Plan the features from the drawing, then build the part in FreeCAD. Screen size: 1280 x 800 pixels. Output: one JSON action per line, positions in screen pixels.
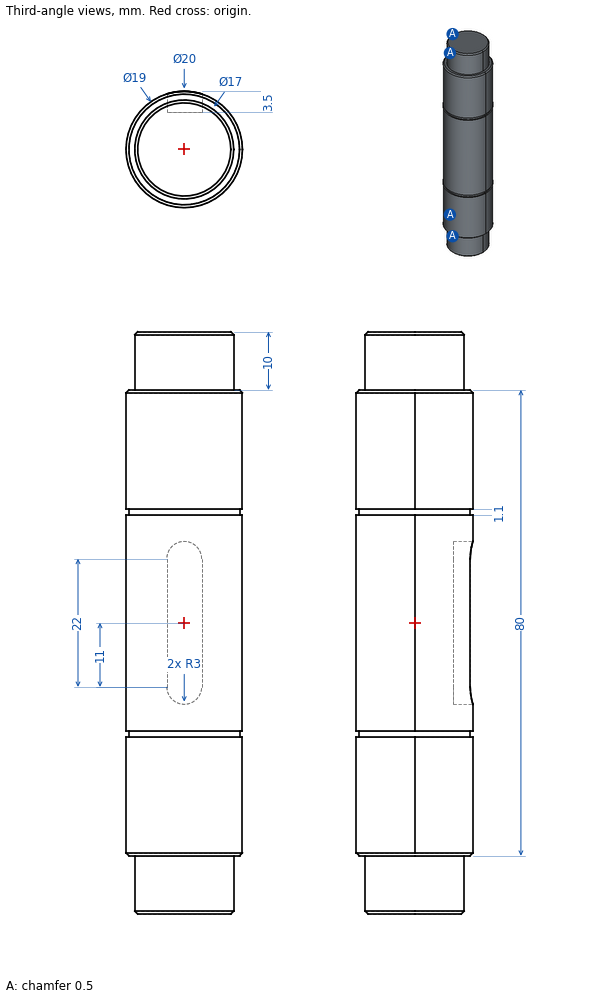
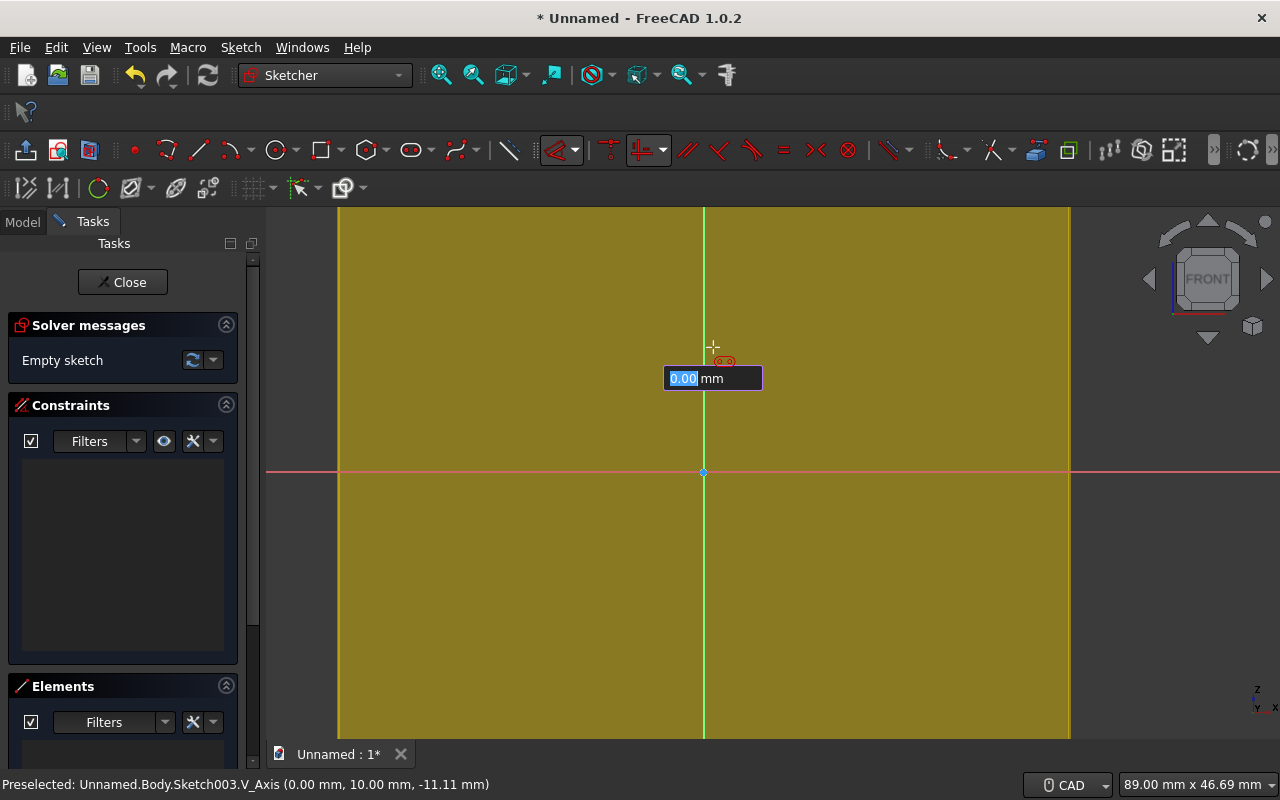
{"action": "left_click", "coordinate": [738, 435]}
{"action": "key", "text": "Escape"}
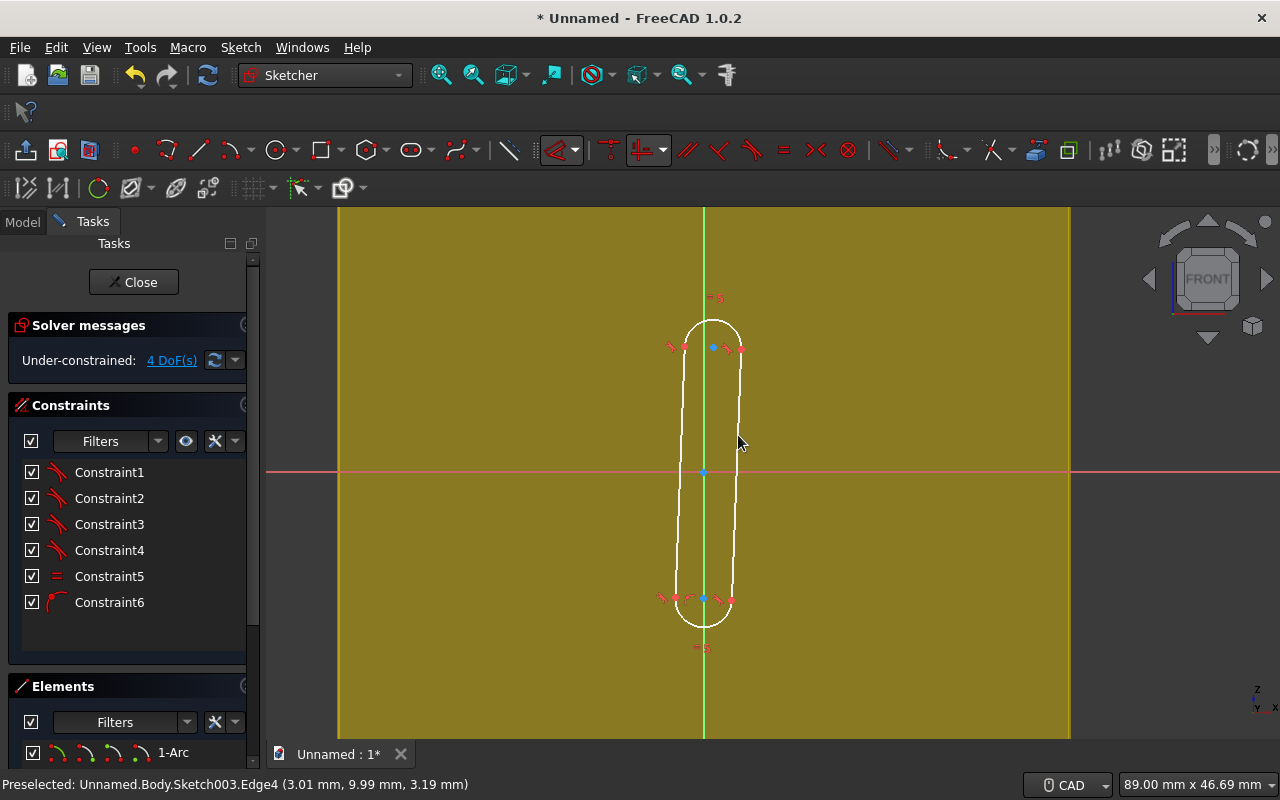
{"action": "left_click", "coordinate": [678, 523]}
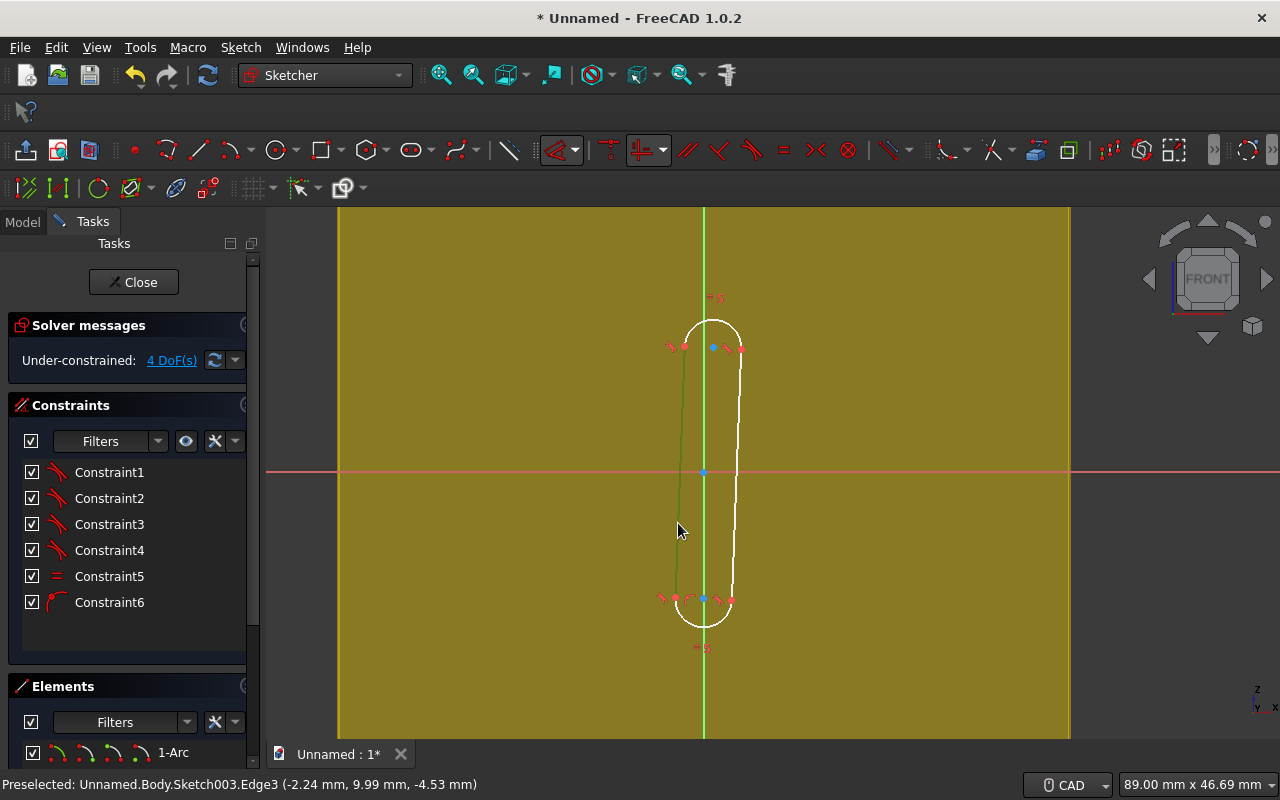
{"action": "left_click", "coordinate": [666, 150]}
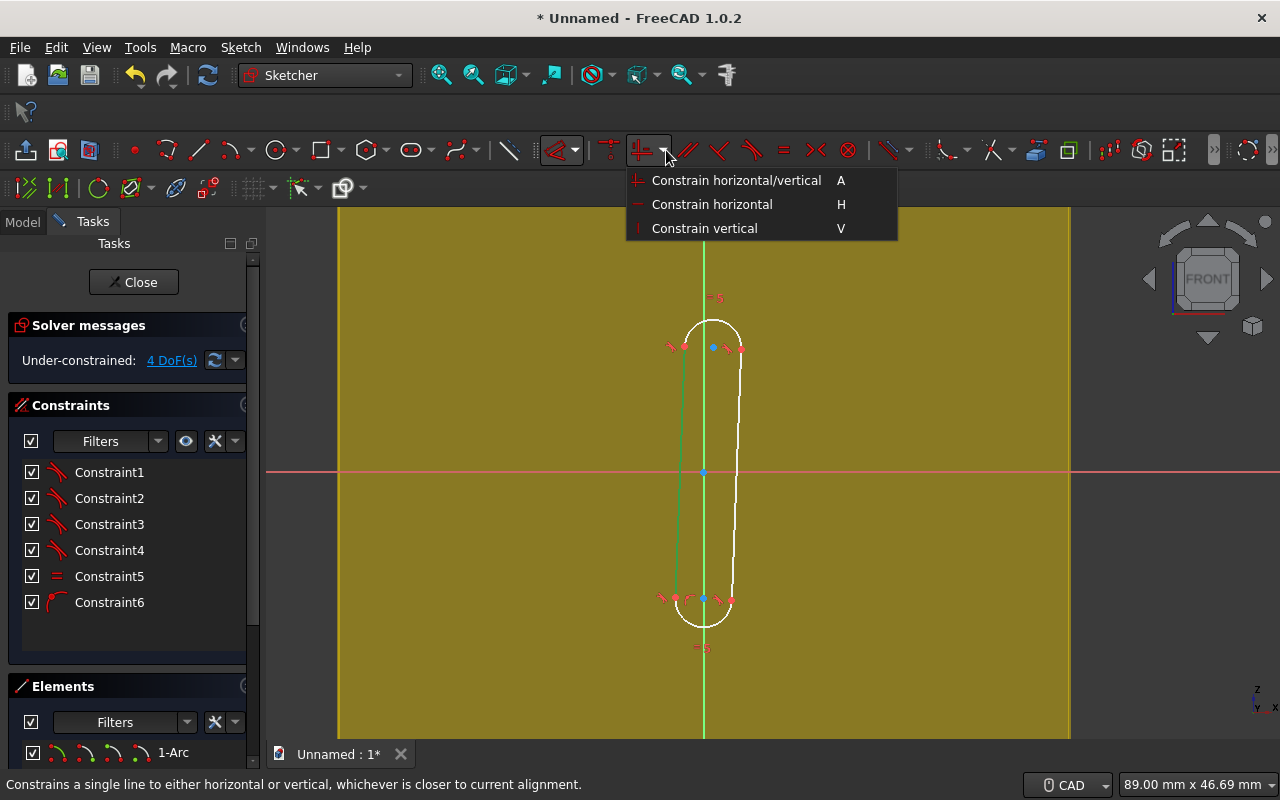
{"action": "left_click", "coordinate": [762, 228]}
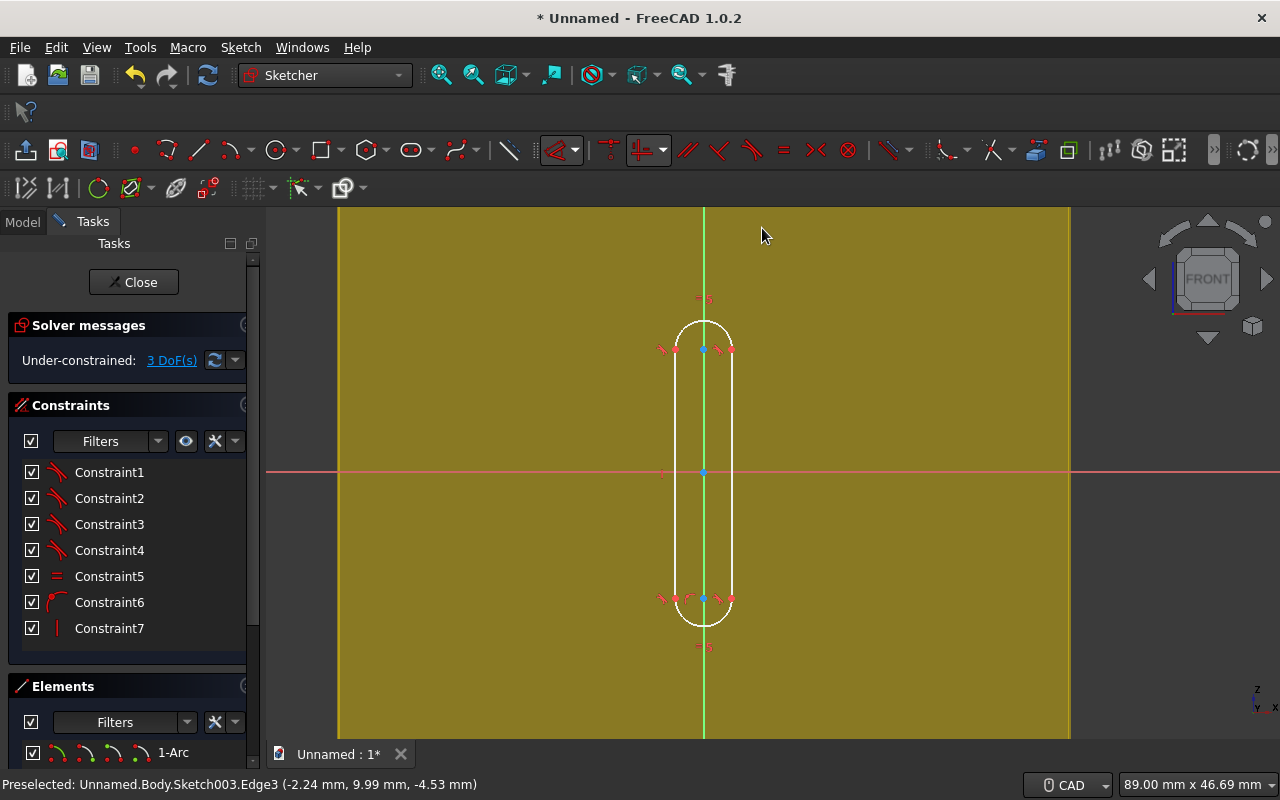
{"action": "key", "text": "d"}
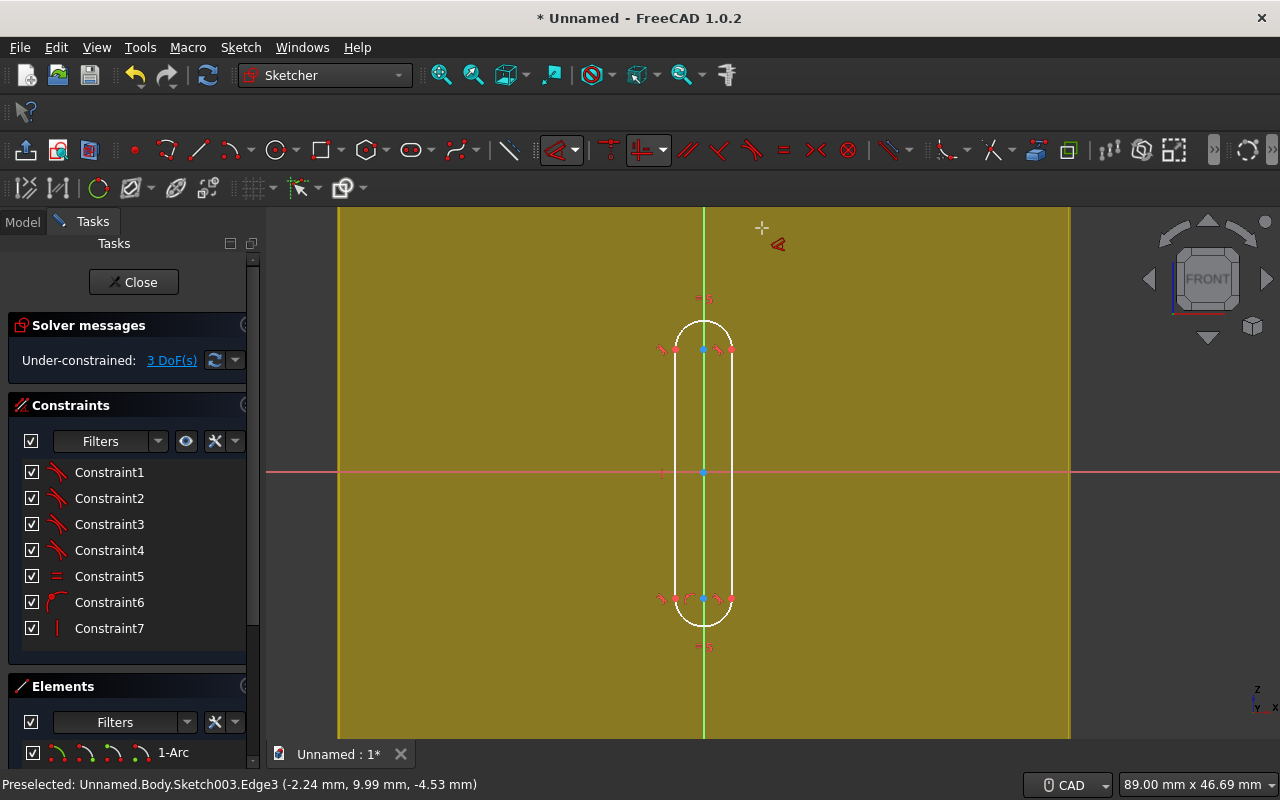
{"action": "left_click", "coordinate": [687, 621]}
{"action": "left_click", "coordinate": [668, 647]}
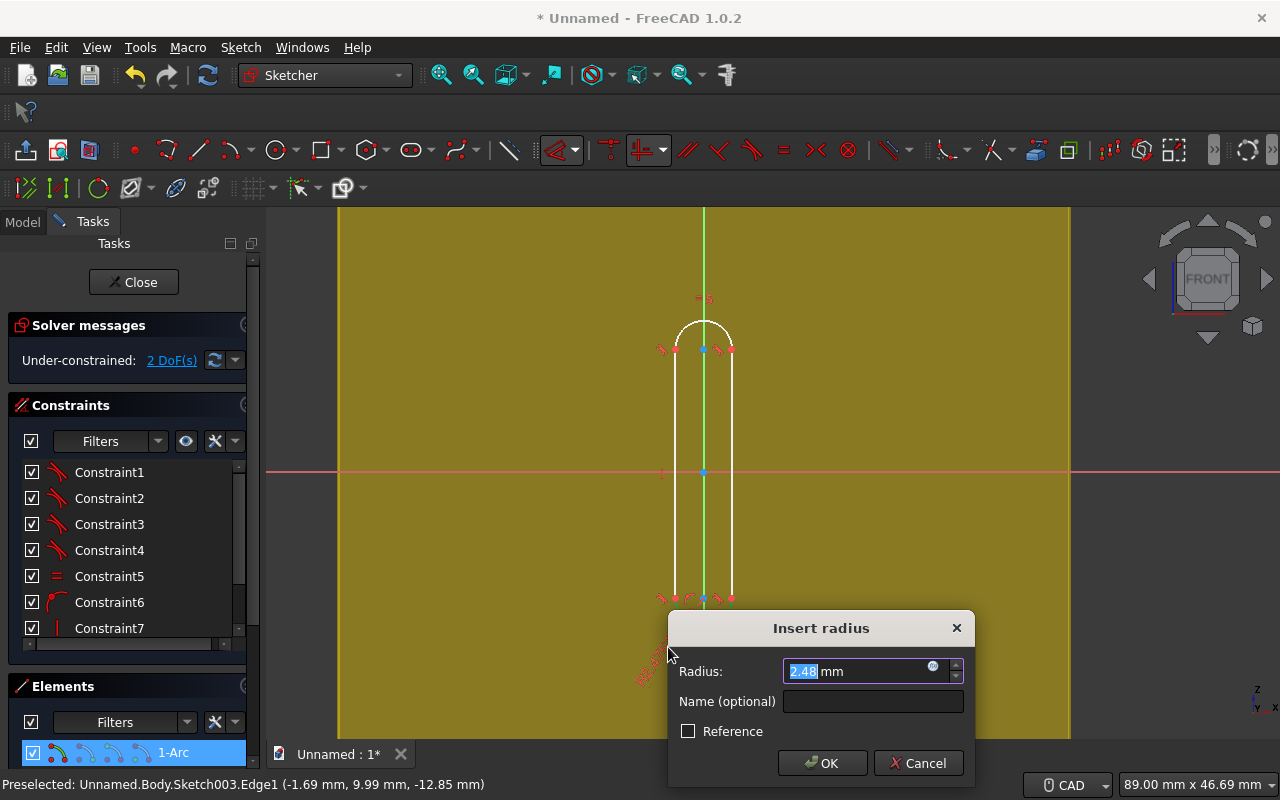
{"action": "type", "text": "3"}
{"action": "key", "text": "Return"}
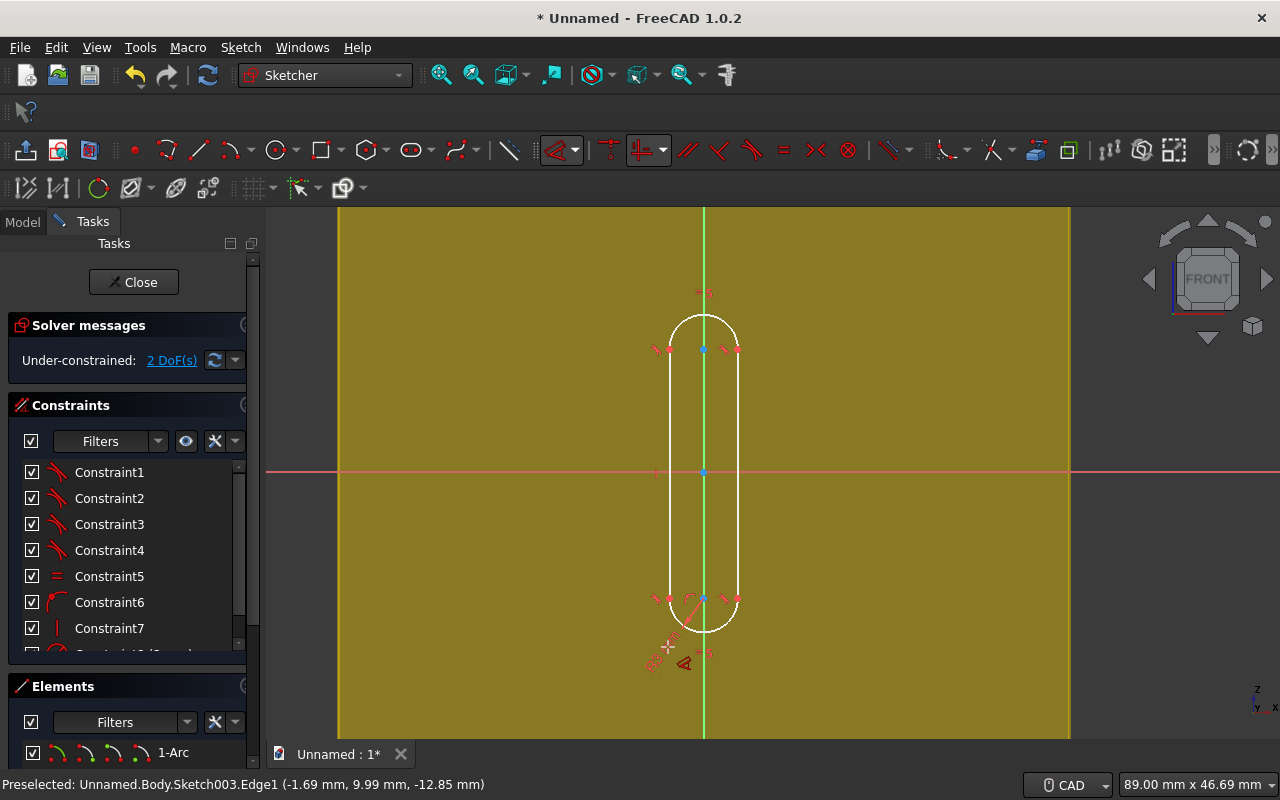
{"action": "left_click", "coordinate": [670, 523]}
{"action": "left_click", "coordinate": [636, 416]}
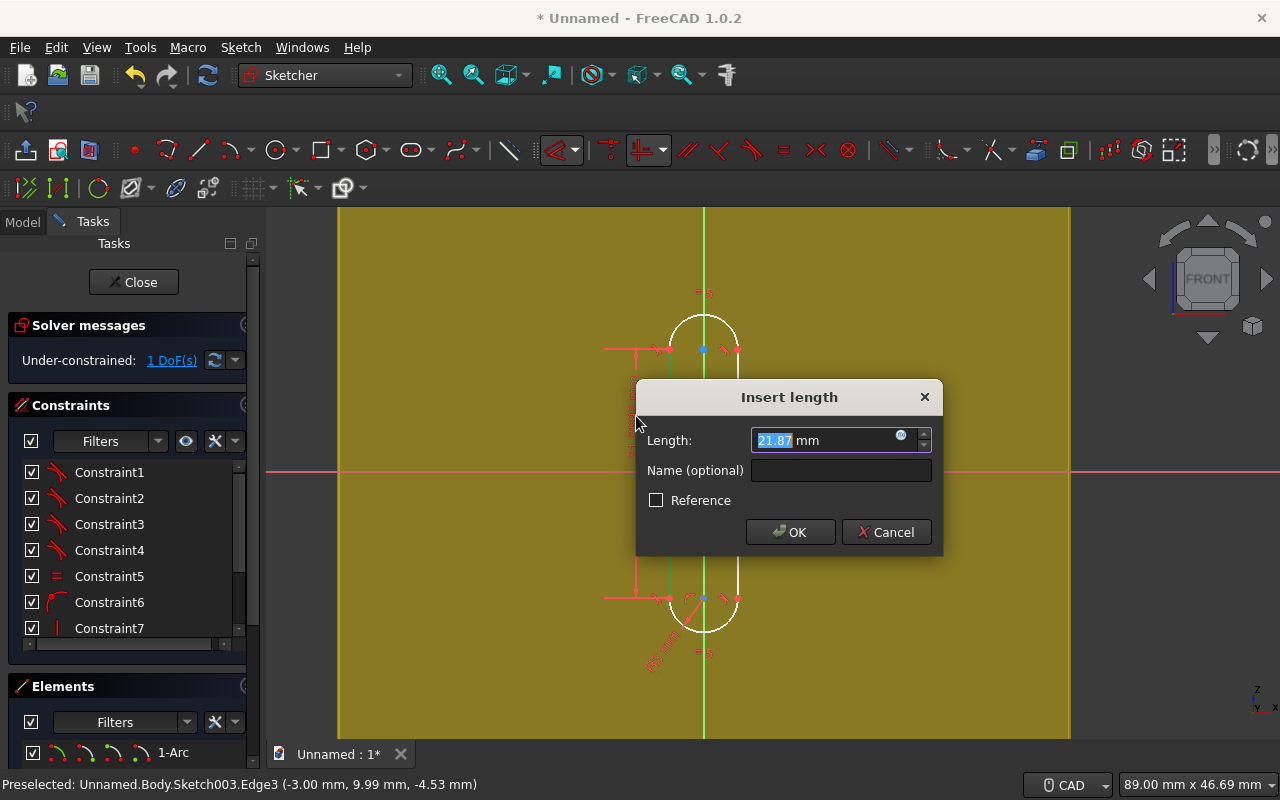
{"action": "type", "text": "22"}
{"action": "key", "text": "Return"}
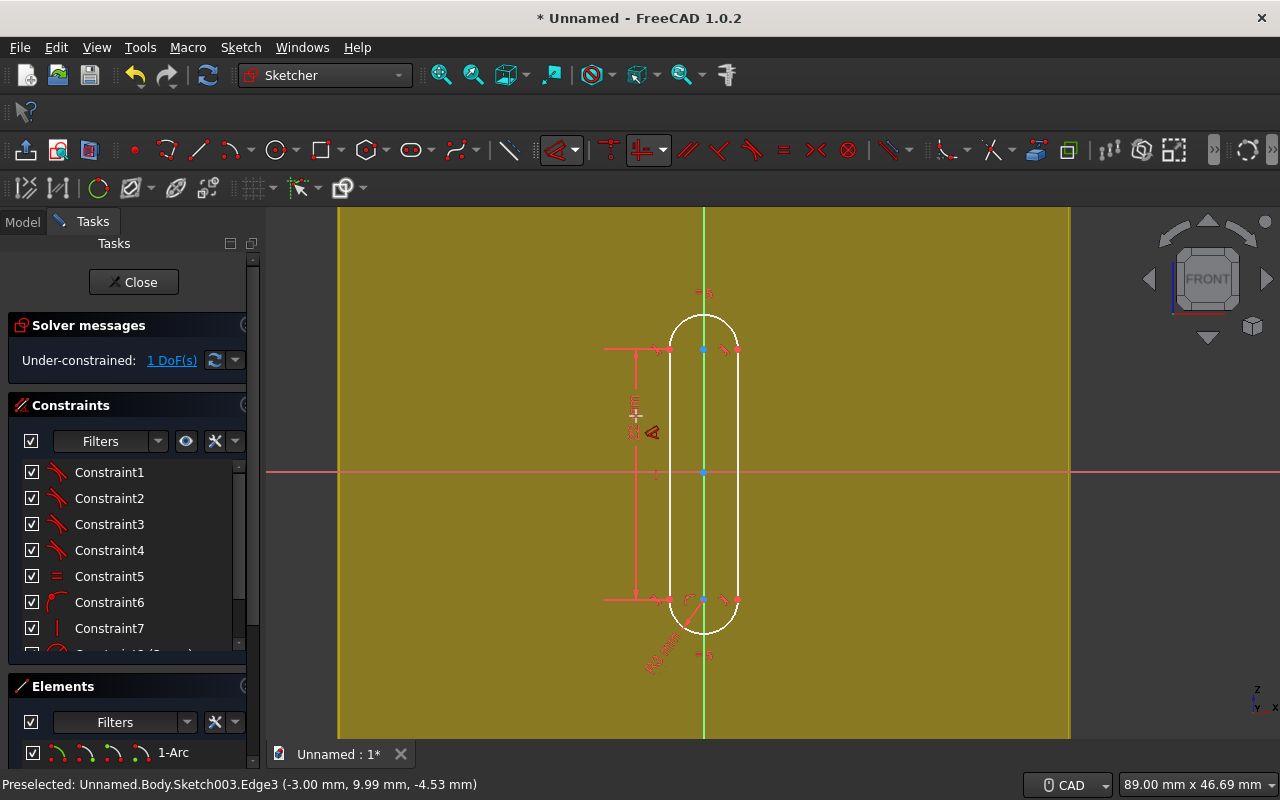
{"action": "left_click", "coordinate": [670, 600]}
{"action": "left_click", "coordinate": [636, 536]}